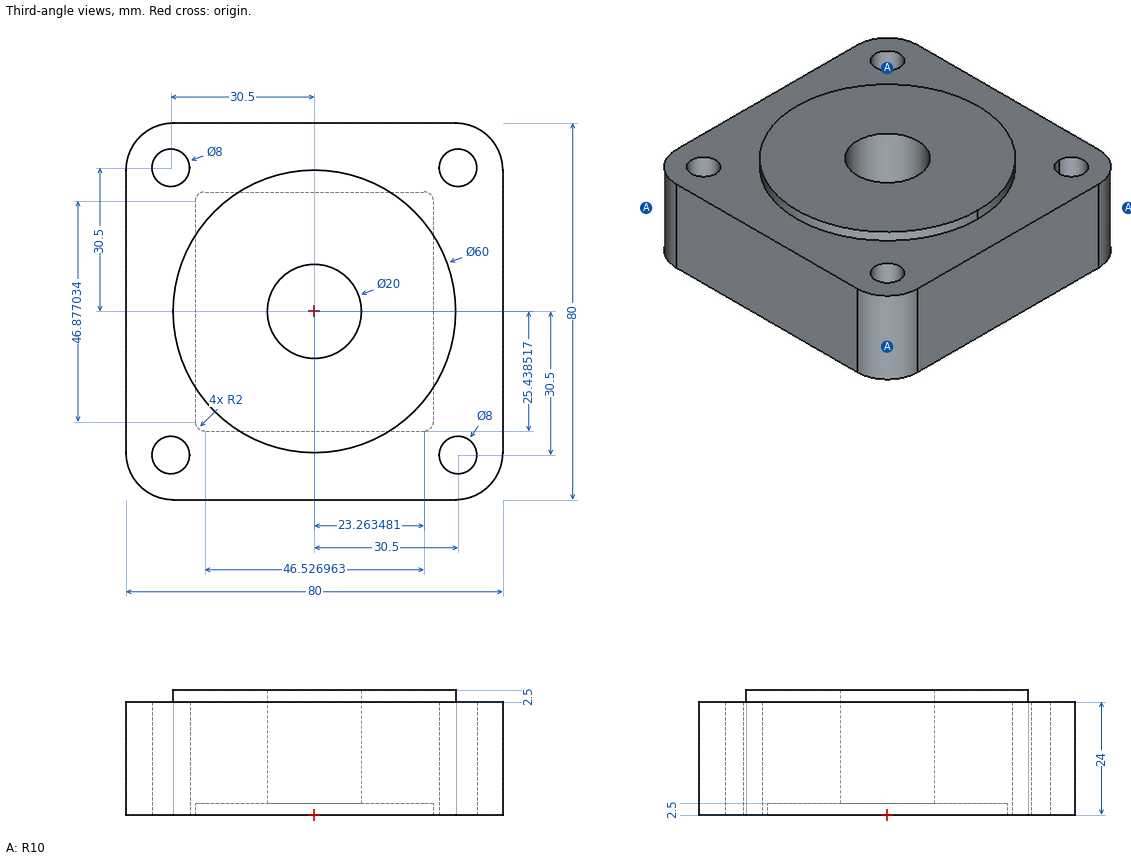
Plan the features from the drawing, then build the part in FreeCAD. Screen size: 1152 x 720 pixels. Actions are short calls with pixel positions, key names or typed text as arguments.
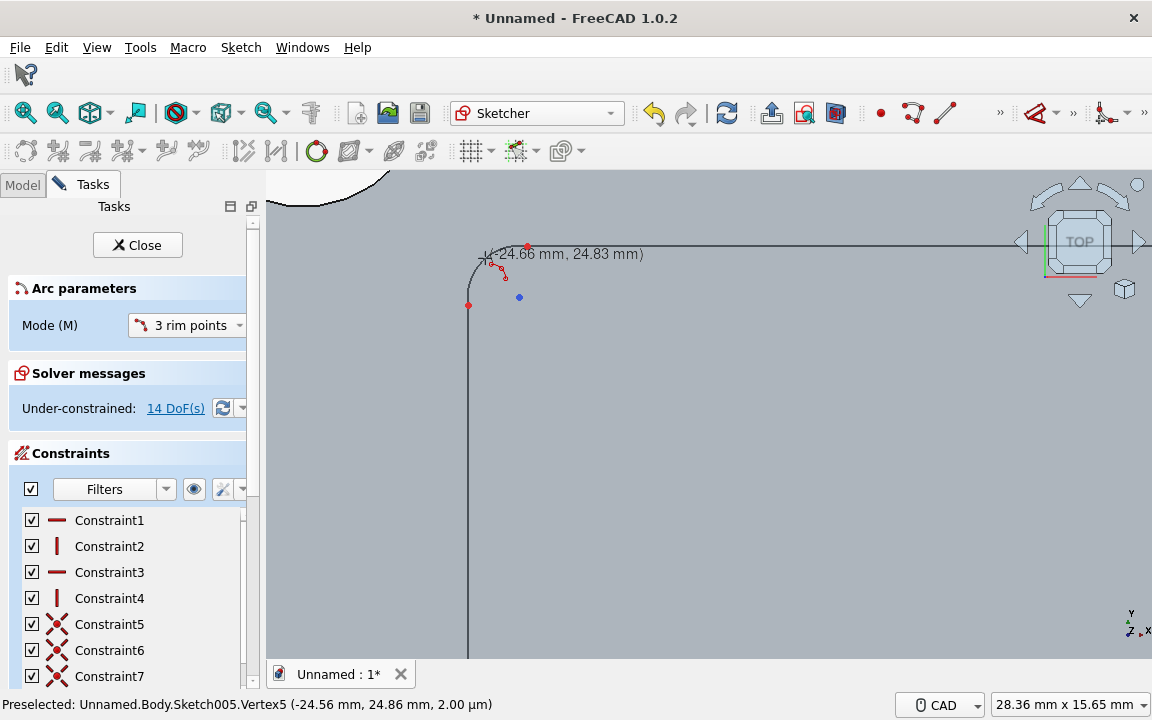
scroll(485, 258, down, 8)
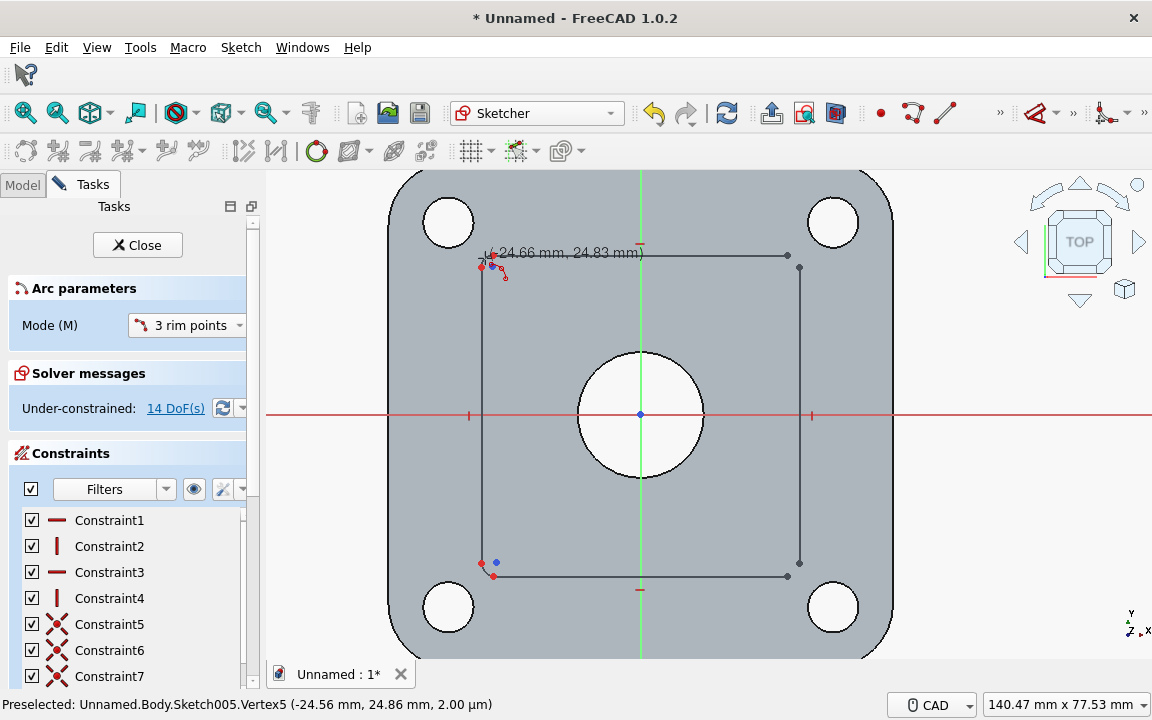
click(788, 256)
click(800, 268)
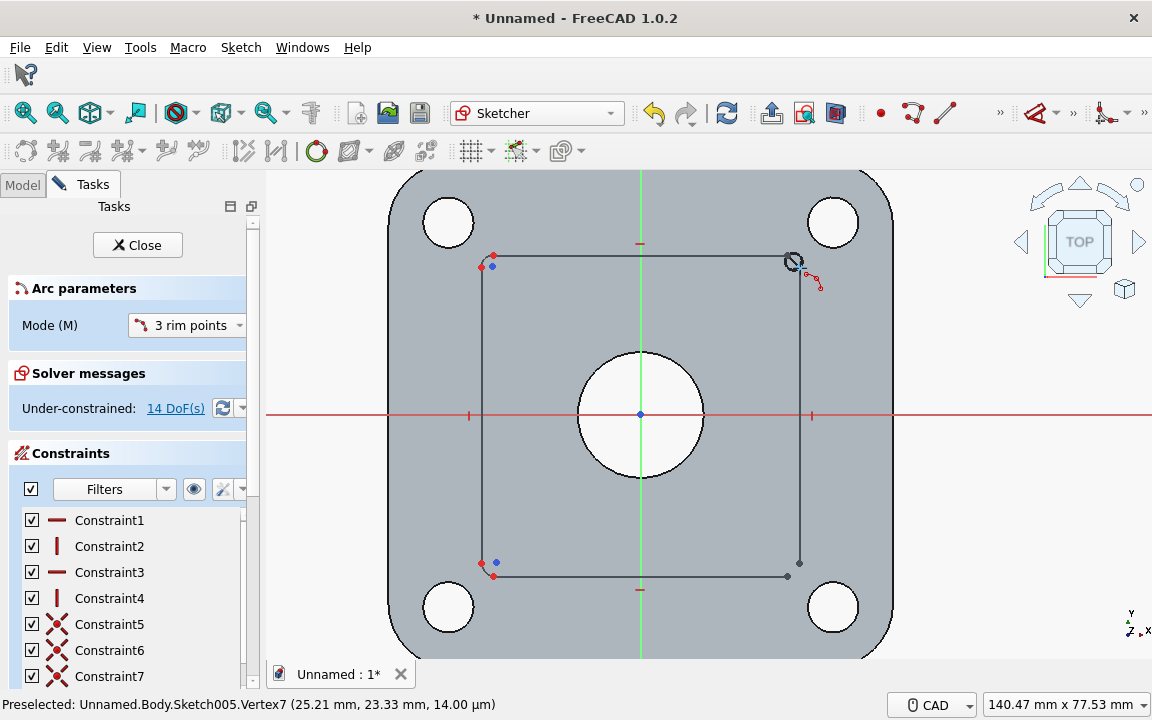
scroll(796, 258, up, 8)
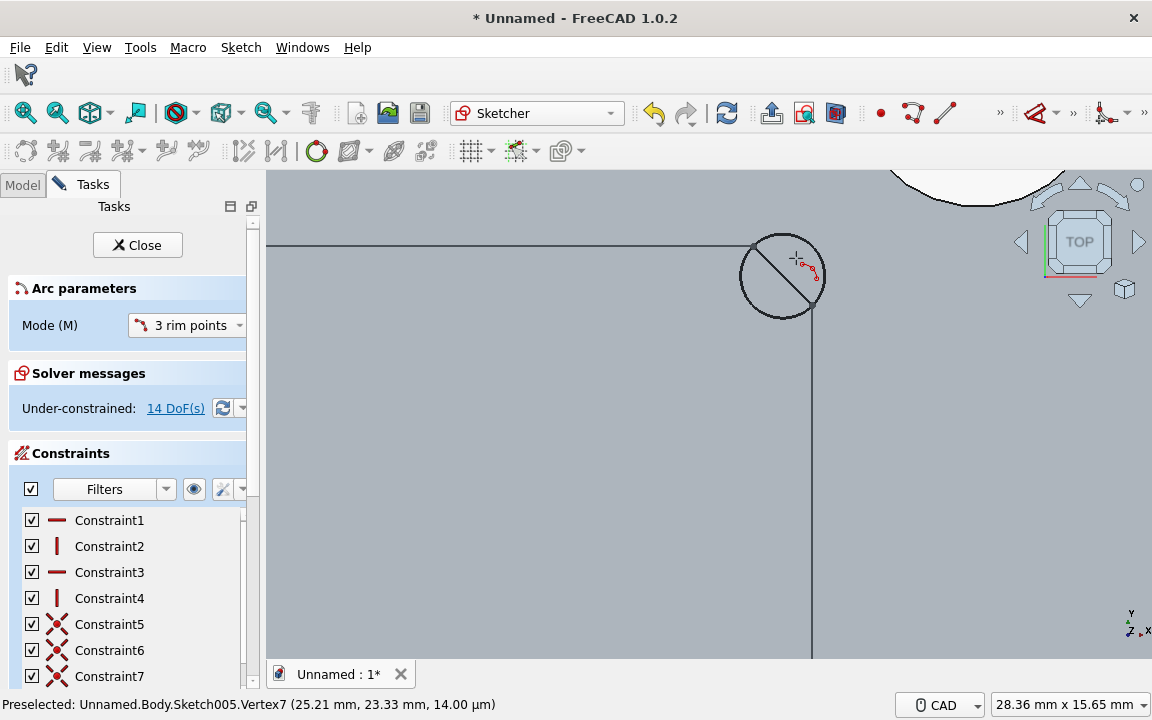
click(796, 258)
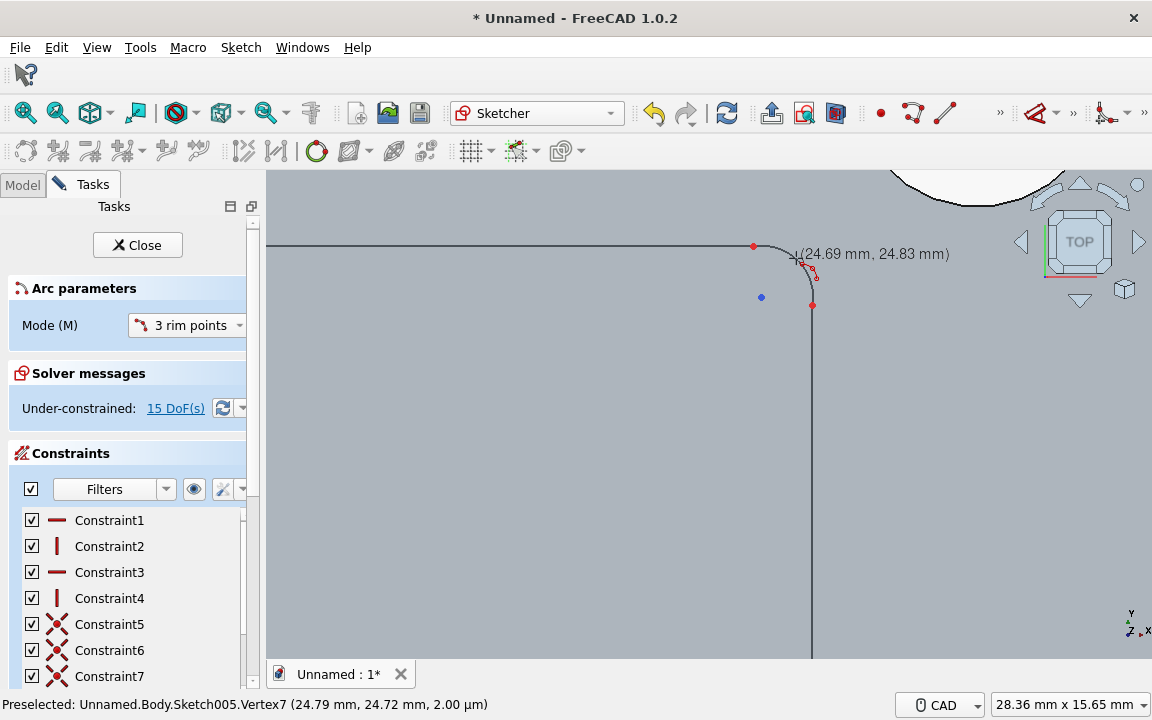
scroll(796, 258, down, 8)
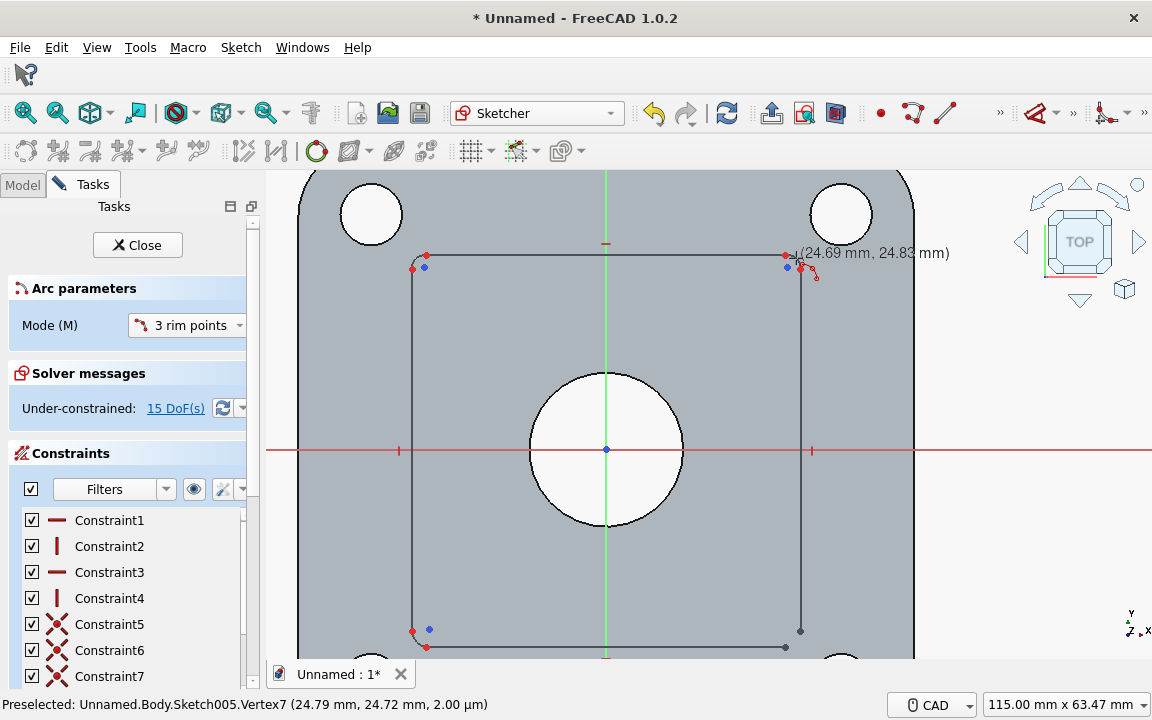
click(800, 564)
click(788, 577)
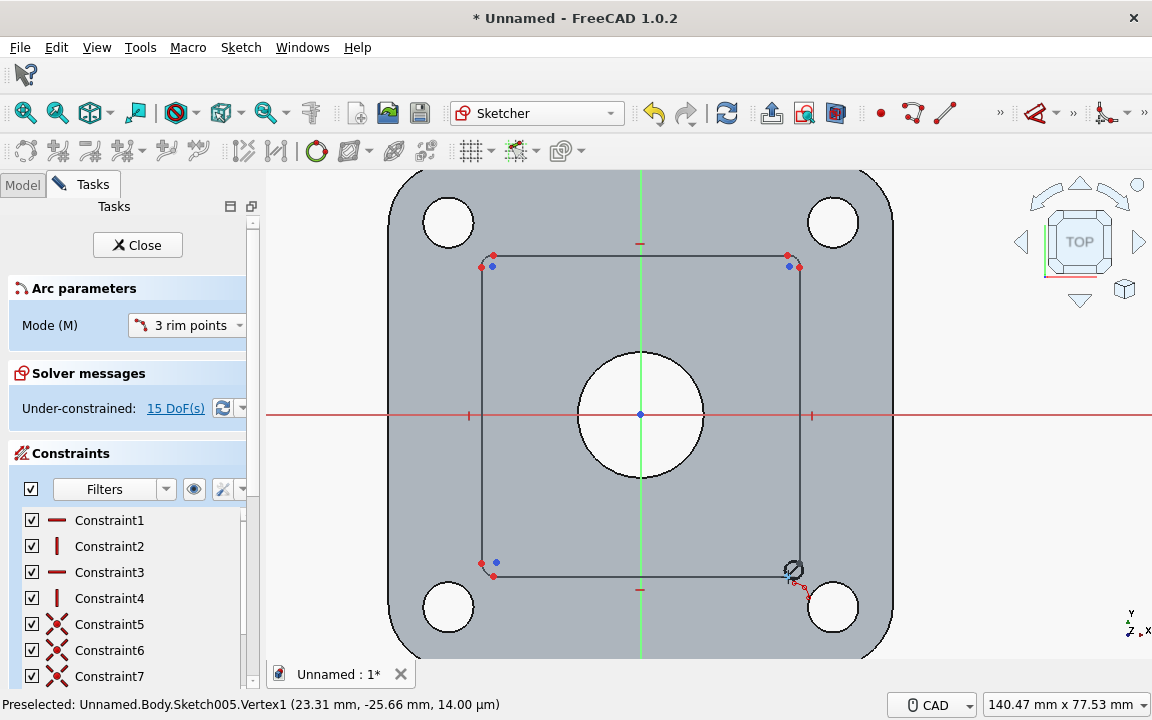
scroll(796, 572, up, 8)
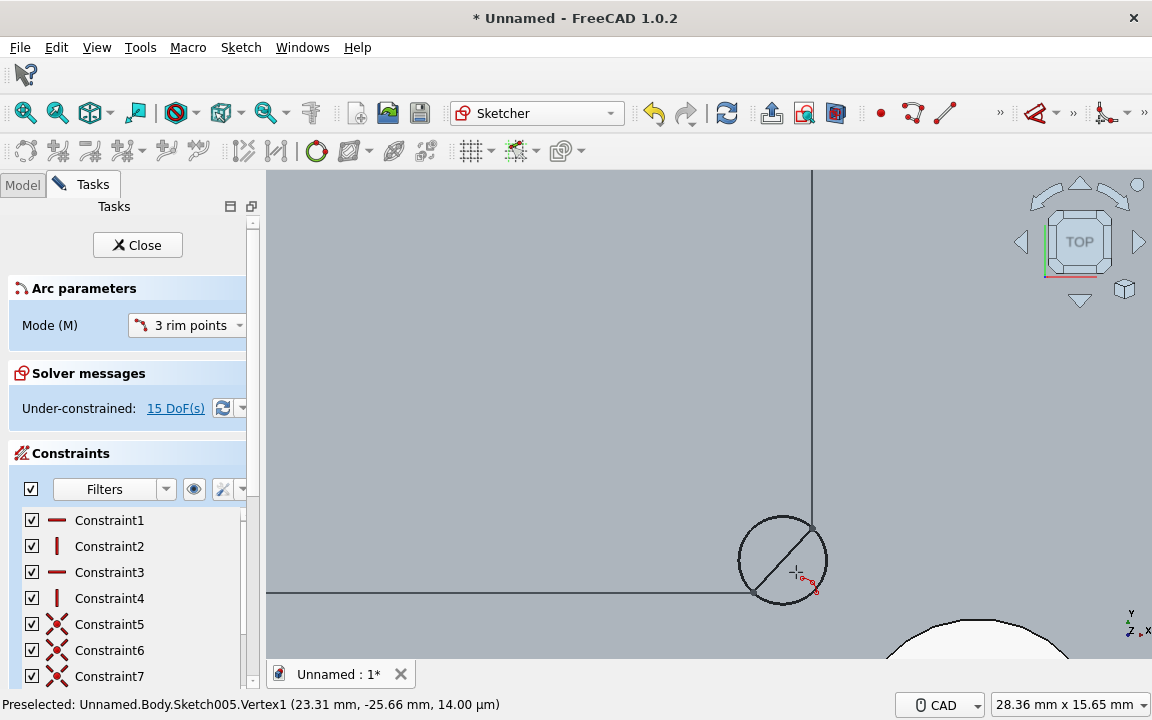
click(796, 567)
key(Escape)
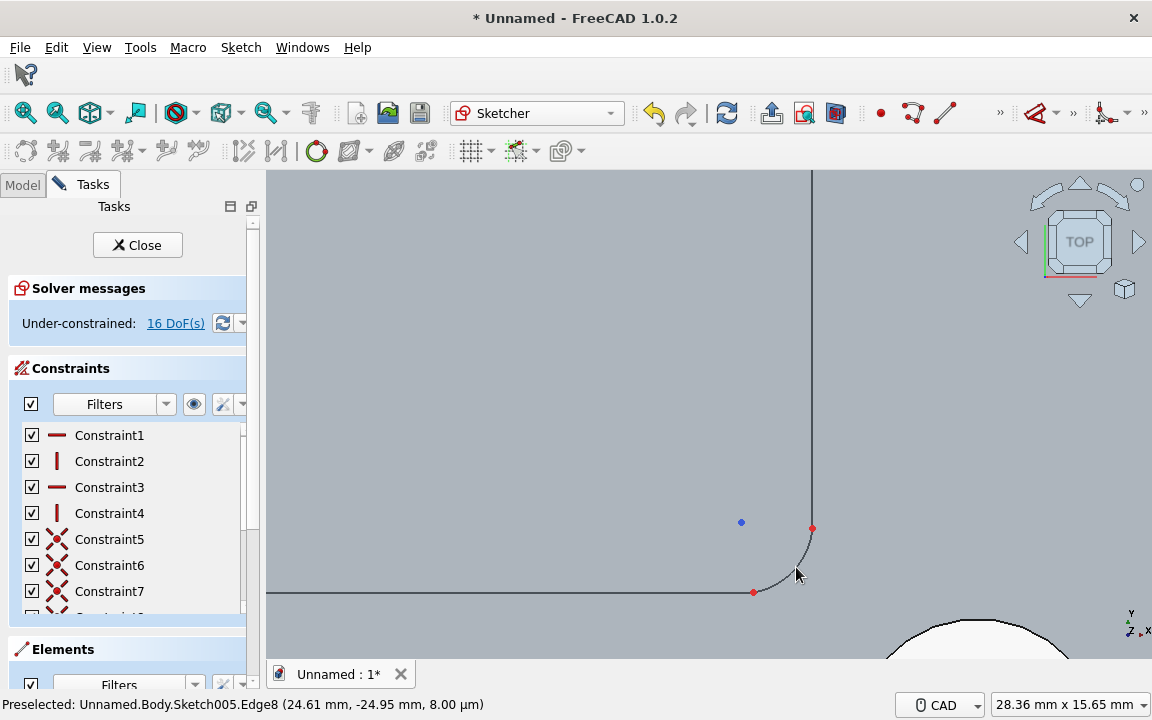
scroll(796, 572, down, 8)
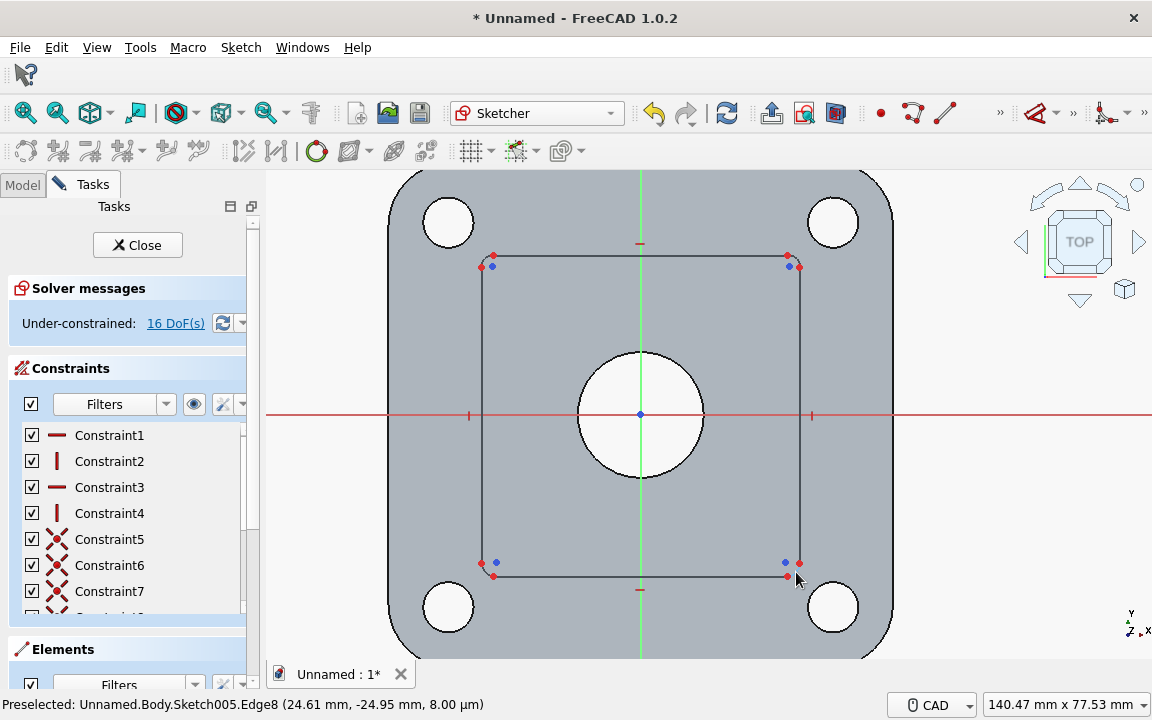
click(700, 577)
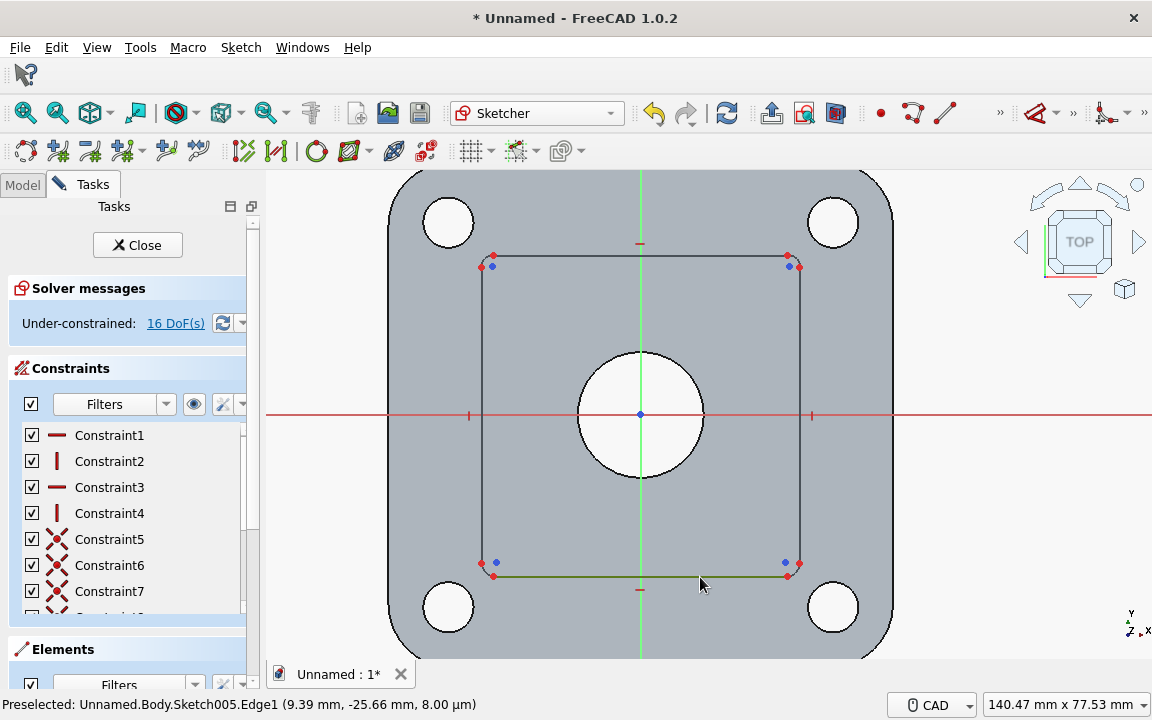
scroll(486, 572, up, 2)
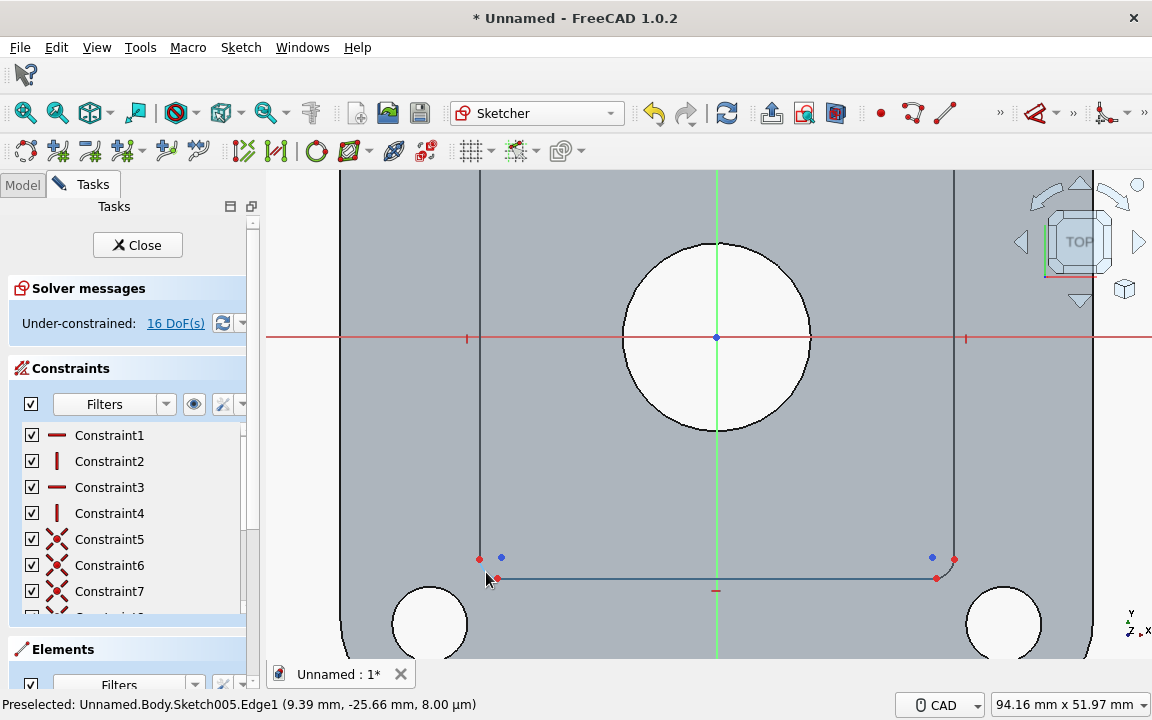
click(485, 572)